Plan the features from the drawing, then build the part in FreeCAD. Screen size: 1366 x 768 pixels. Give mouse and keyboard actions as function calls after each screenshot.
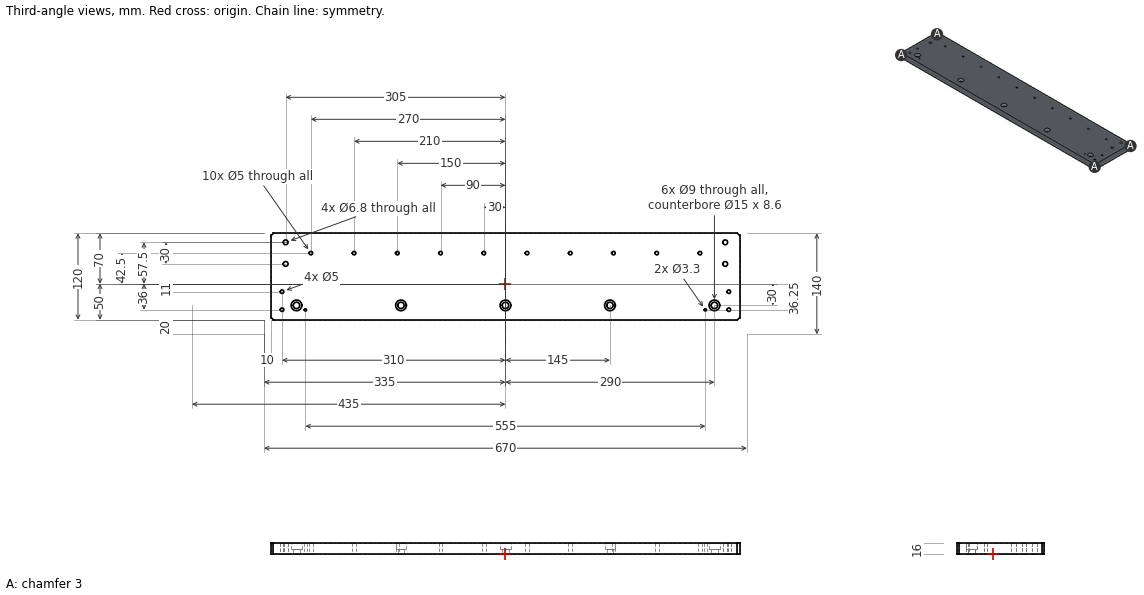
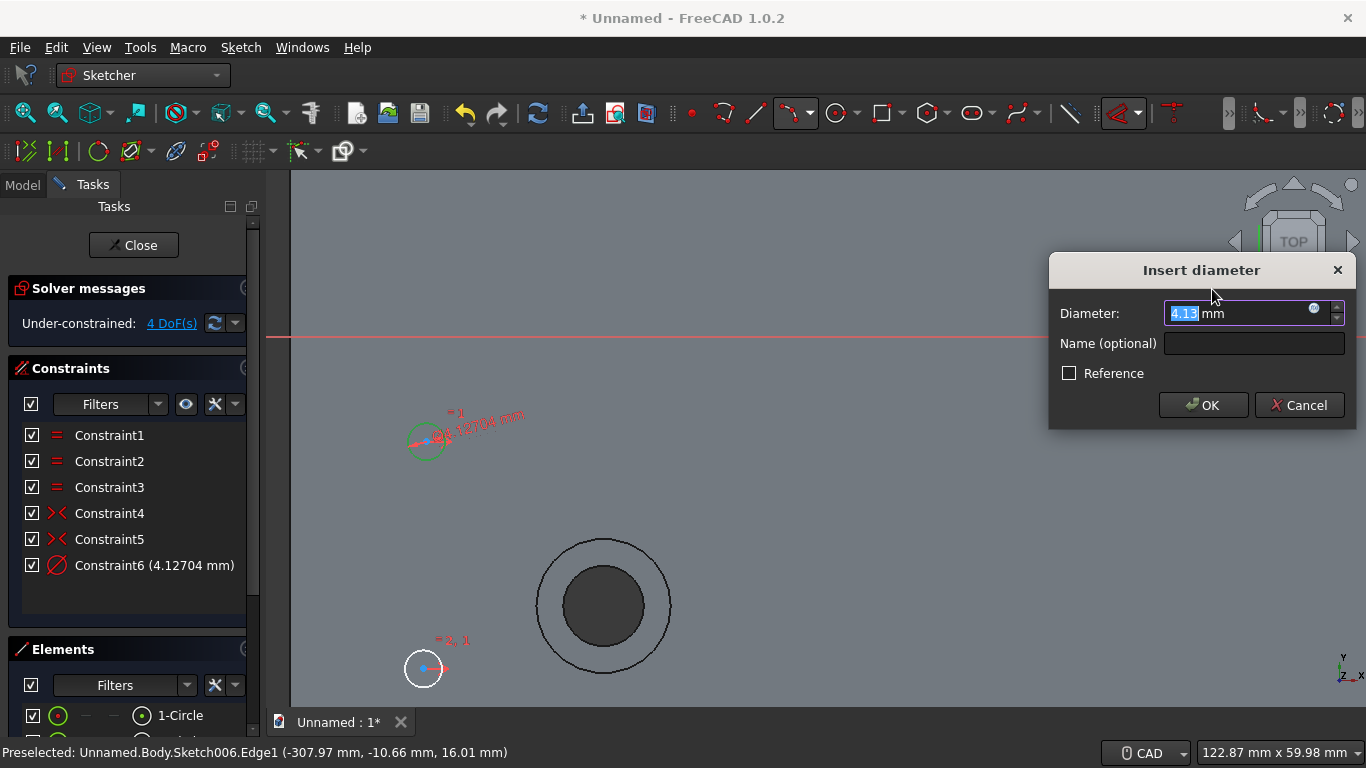
text(5)
key(Return)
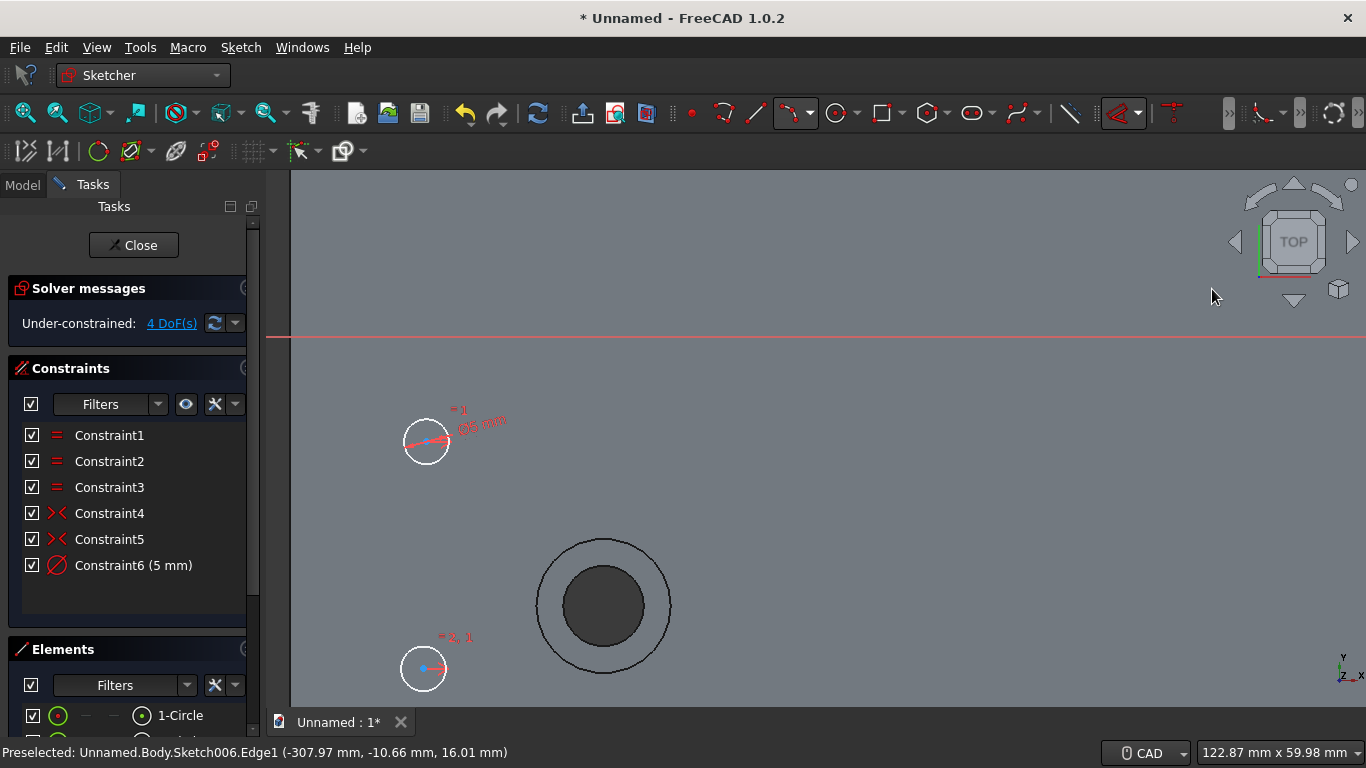
click(426, 442)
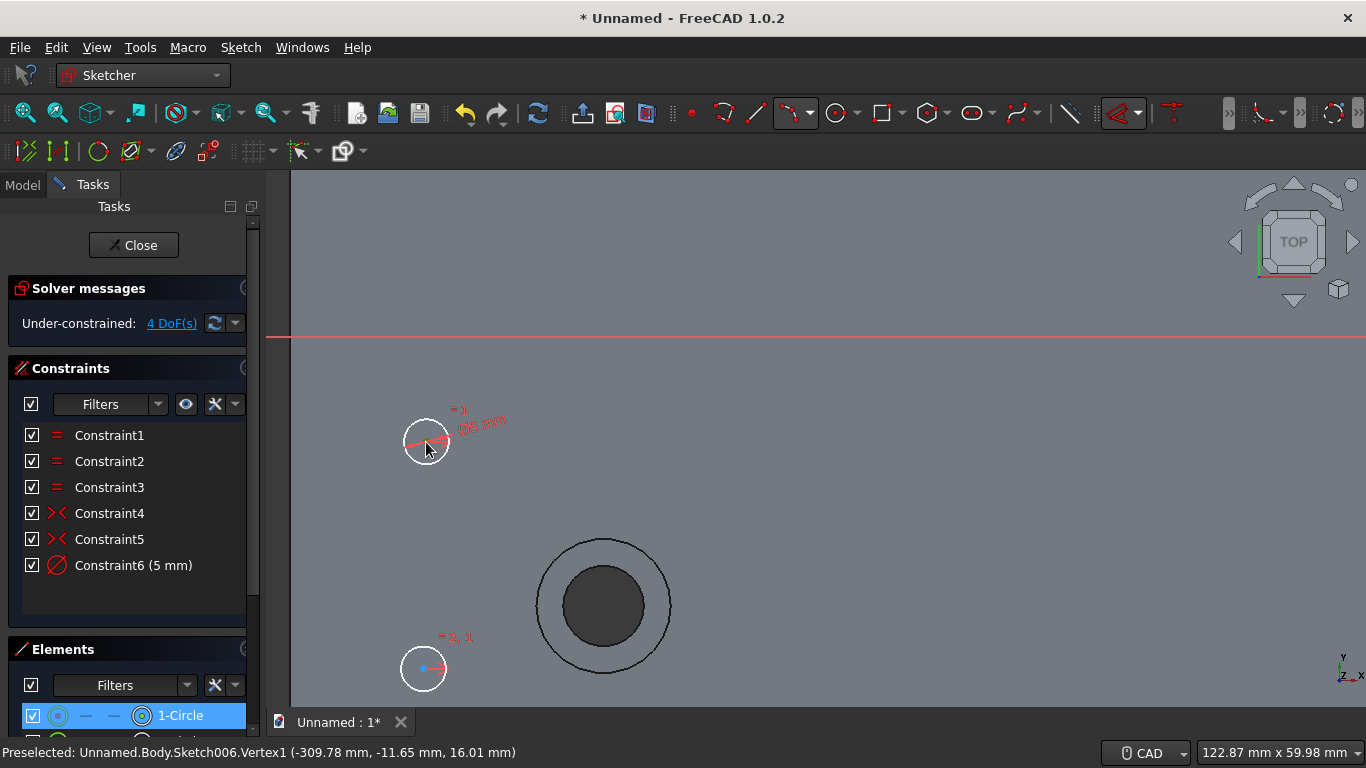
click(1140, 114)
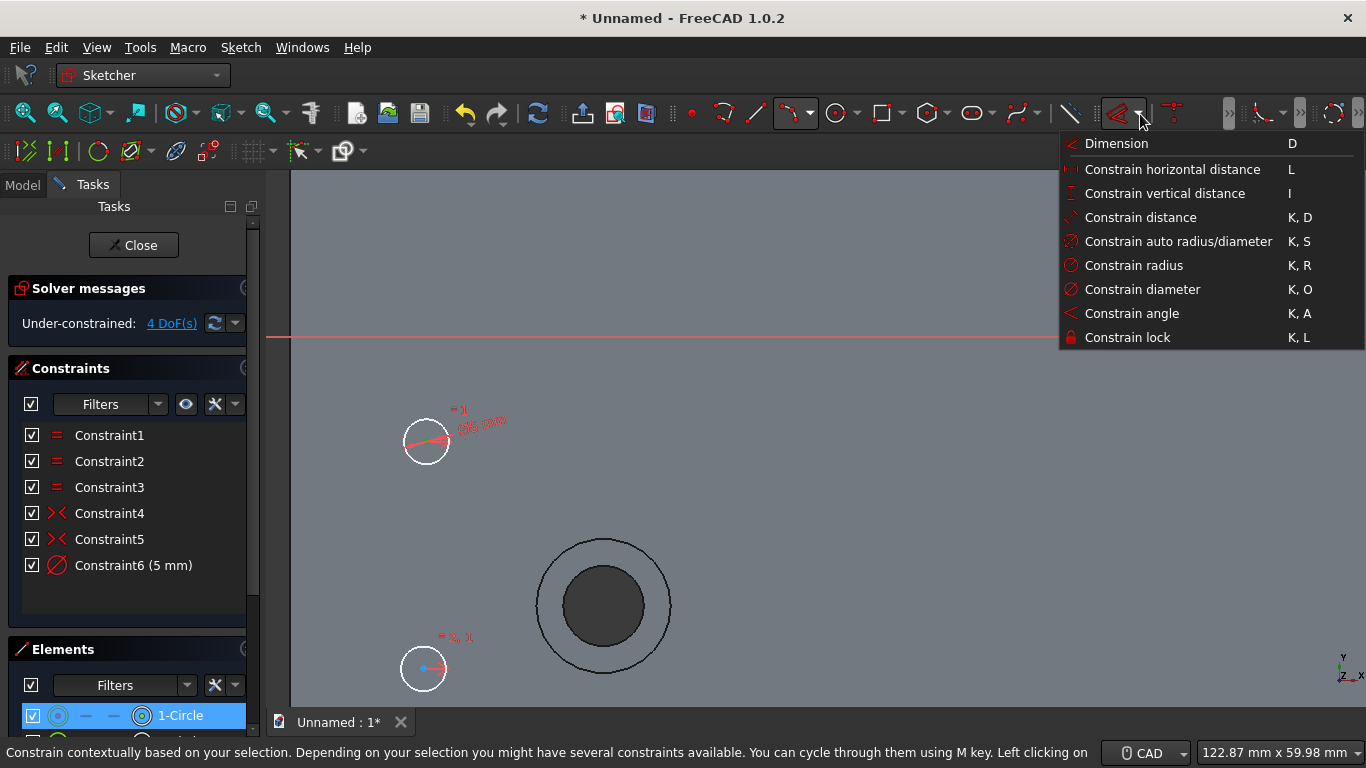
click(1212, 193)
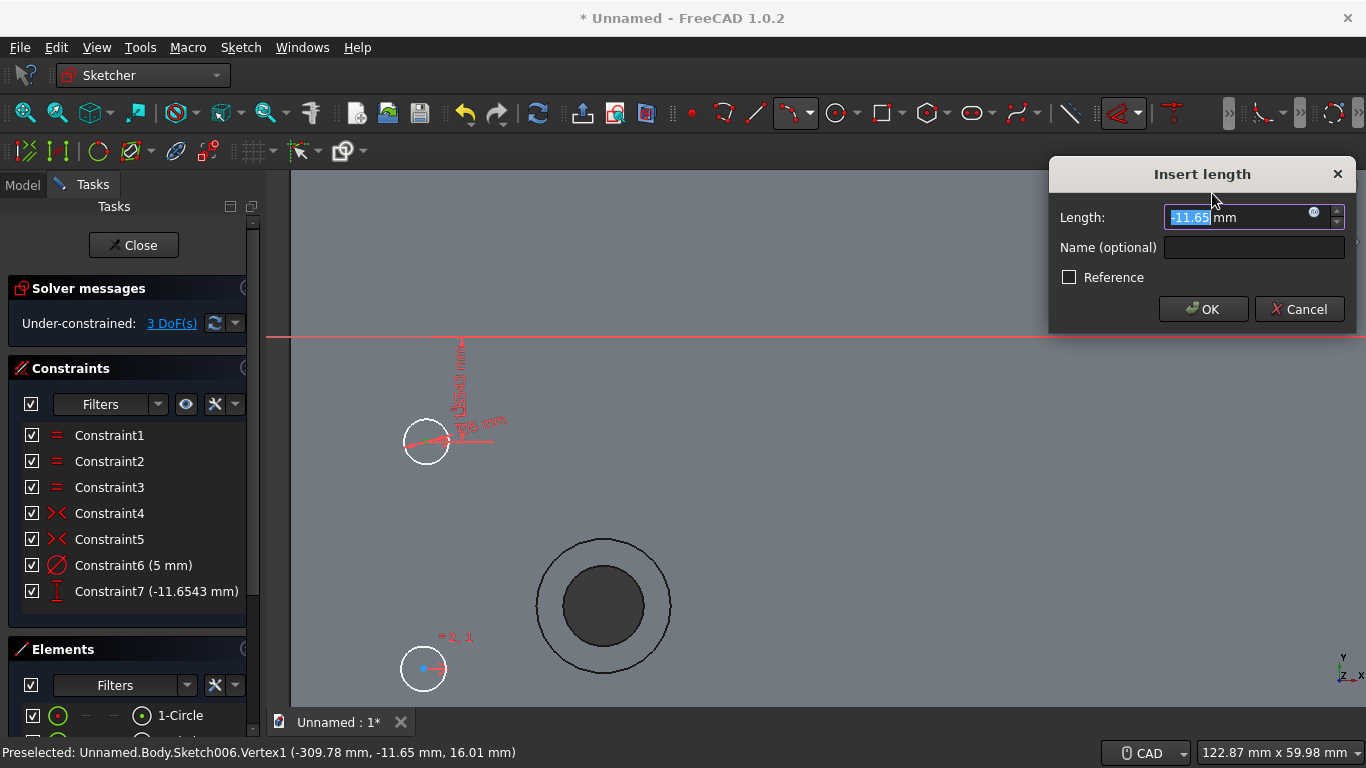
text(-11)
key(Return)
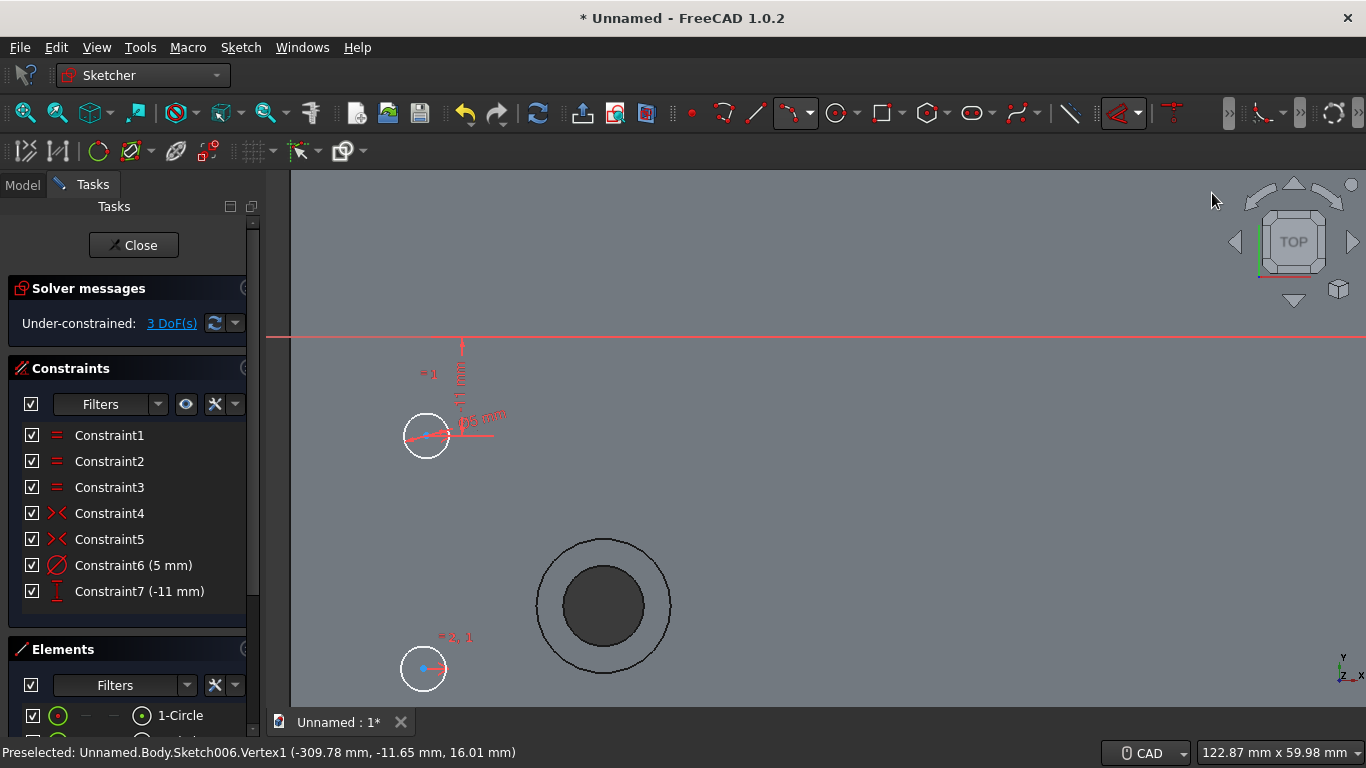
scroll(442, 430, down, 11)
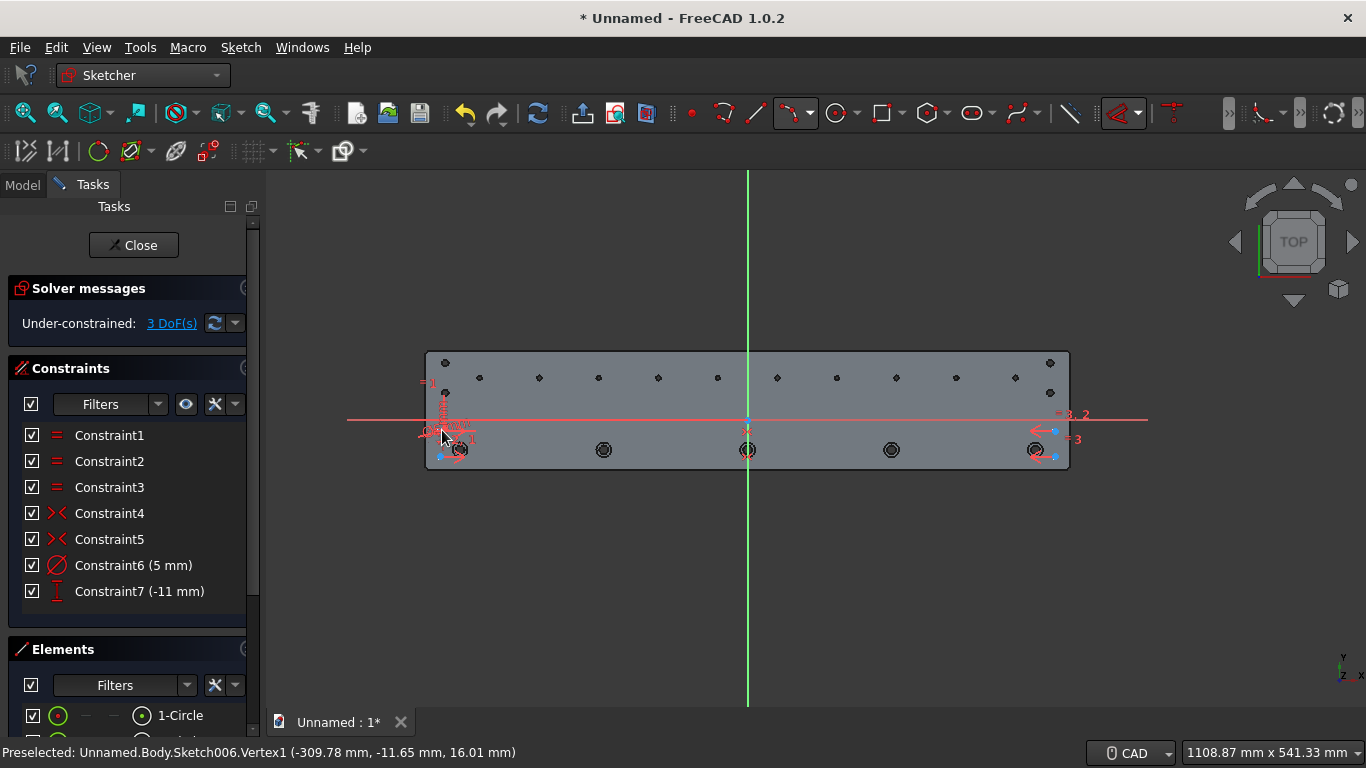
click(440, 457)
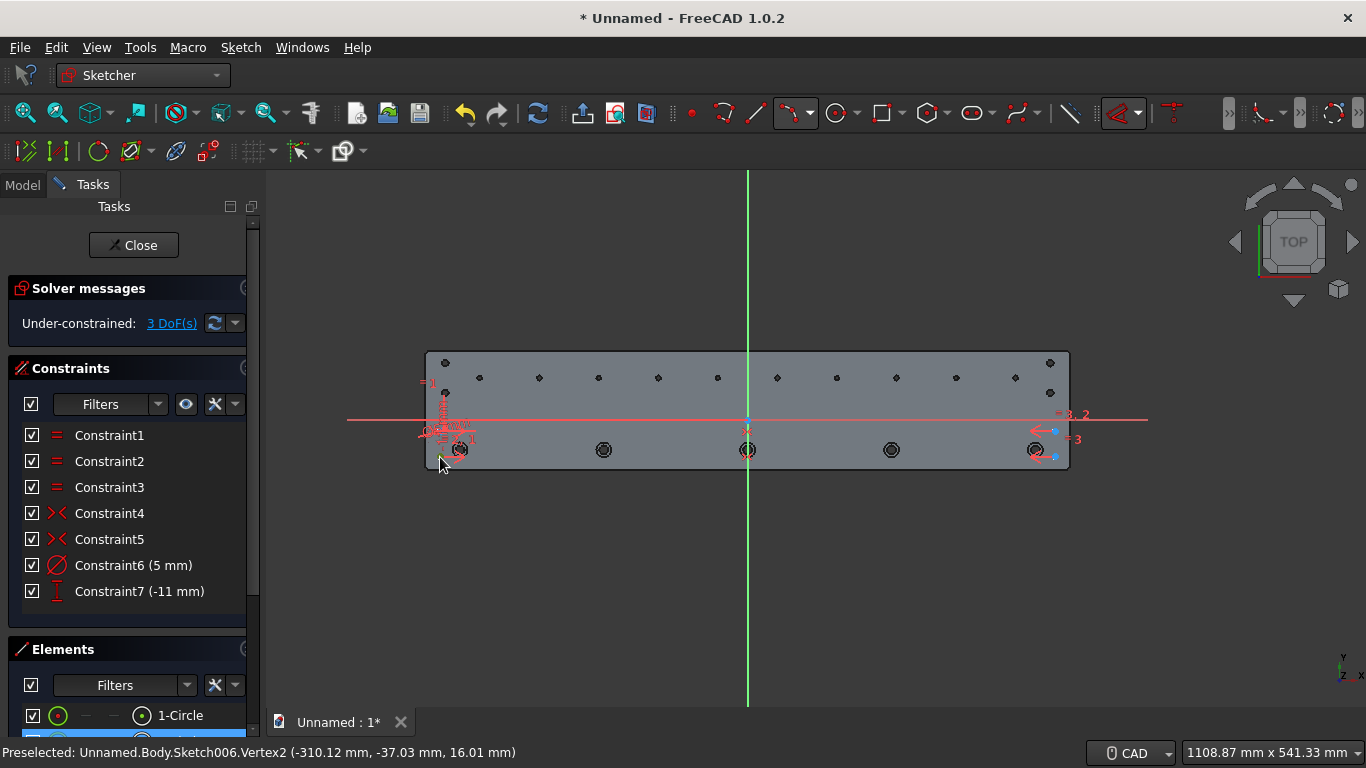
click(1140, 114)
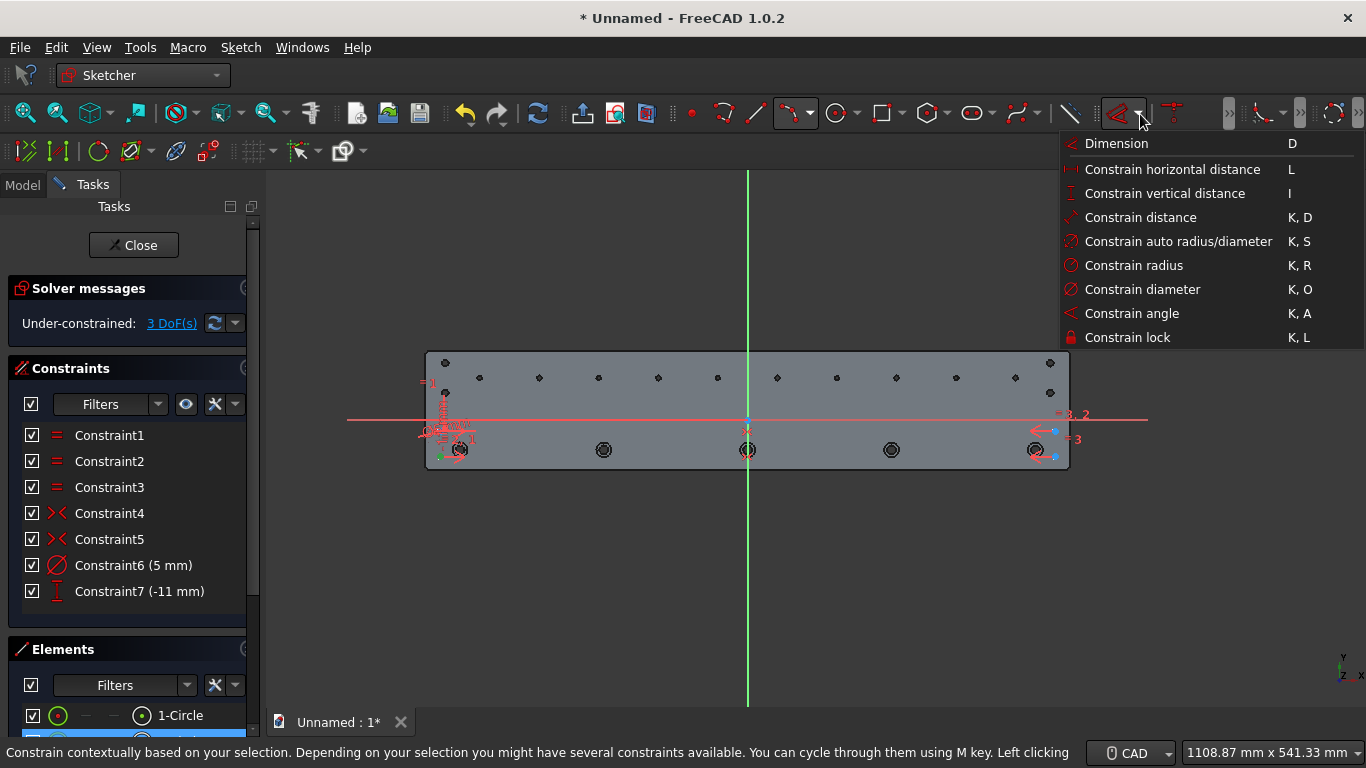
click(1212, 193)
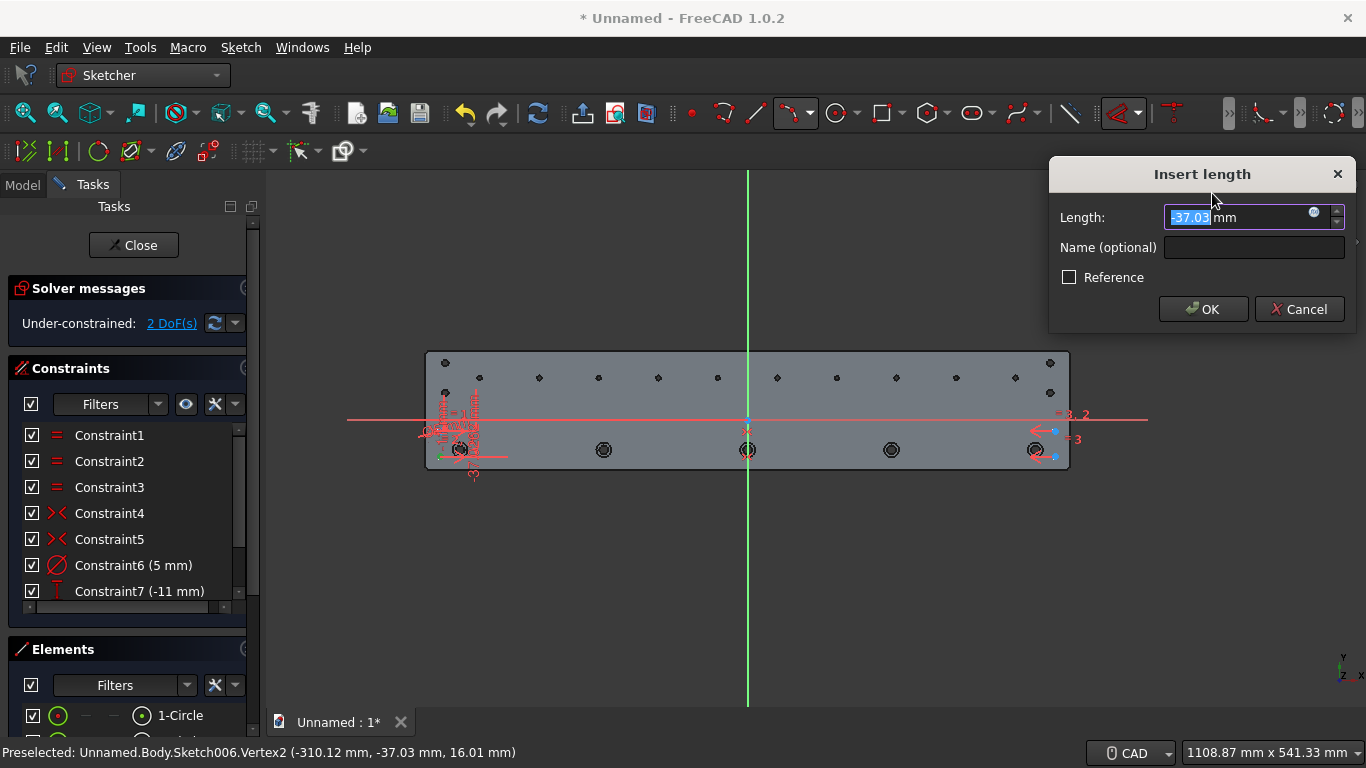
text(-36)
key(Return)